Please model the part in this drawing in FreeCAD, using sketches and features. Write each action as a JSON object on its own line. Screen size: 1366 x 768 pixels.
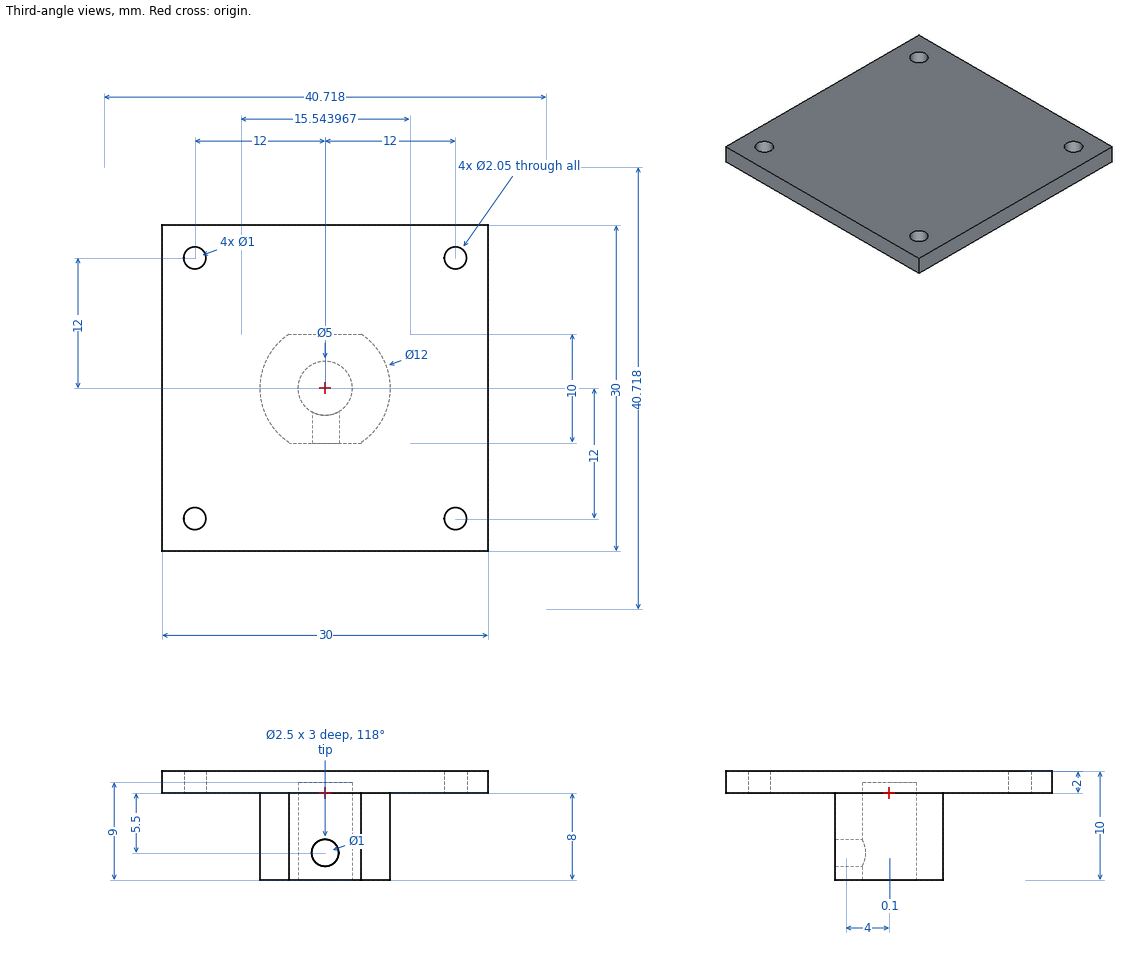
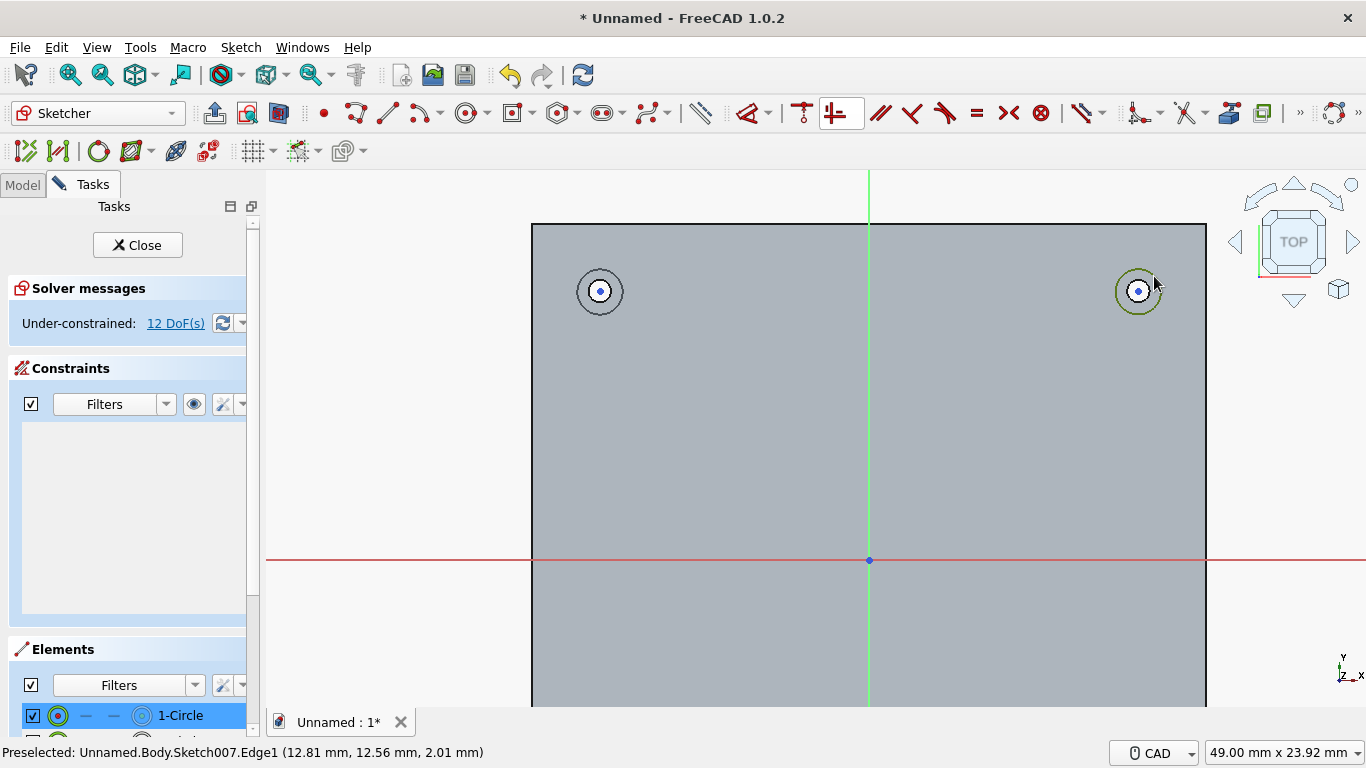
{"action": "scroll", "coordinate": [600, 290], "scroll_direction": "down", "scroll_amount": 3}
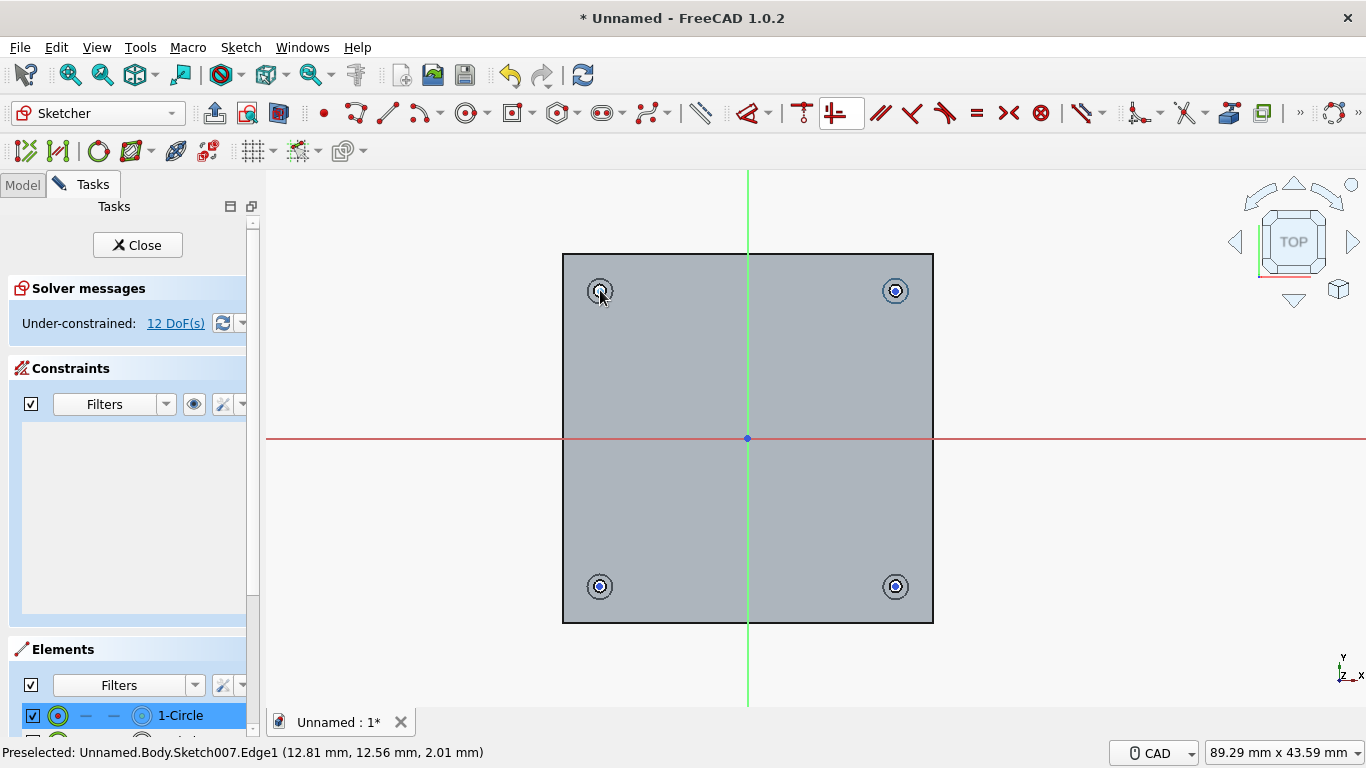
{"action": "left_click", "coordinate": [904, 578]}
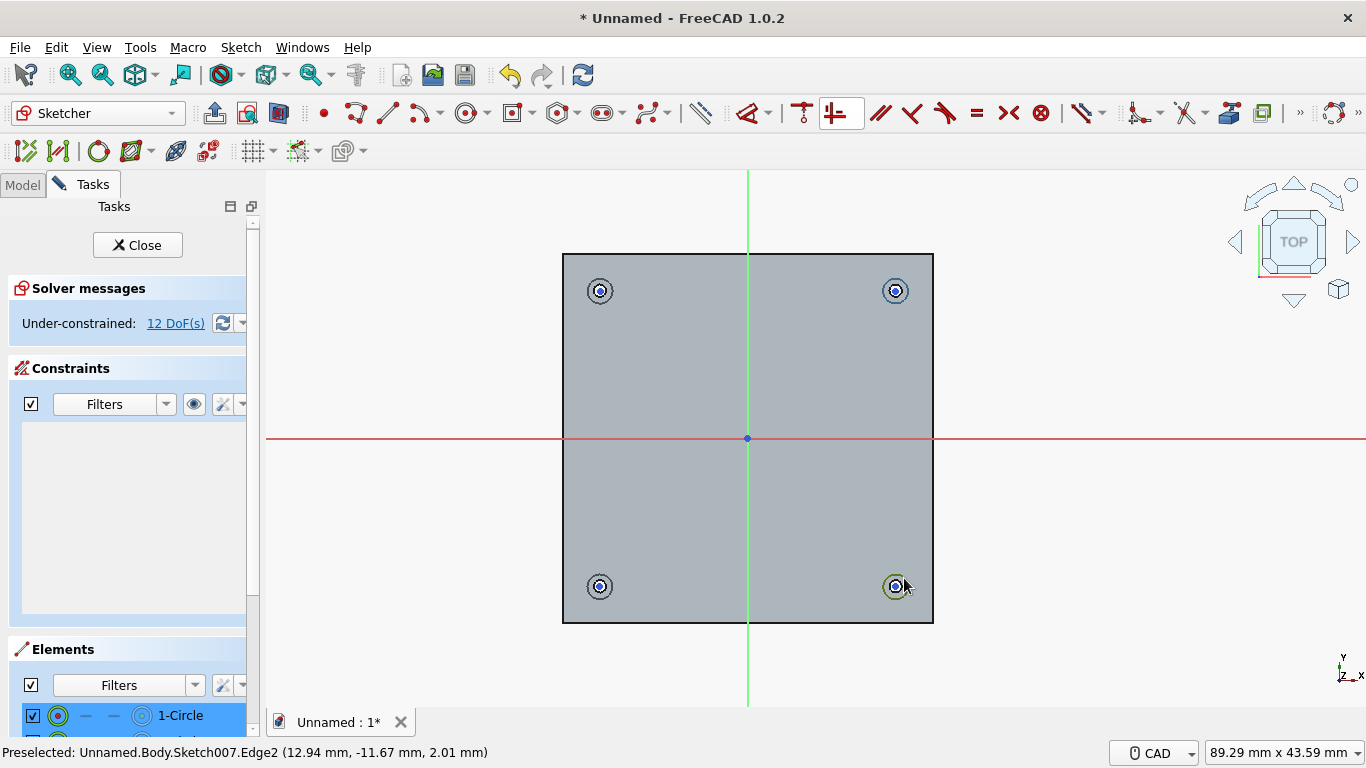
{"action": "left_click", "coordinate": [609, 578]}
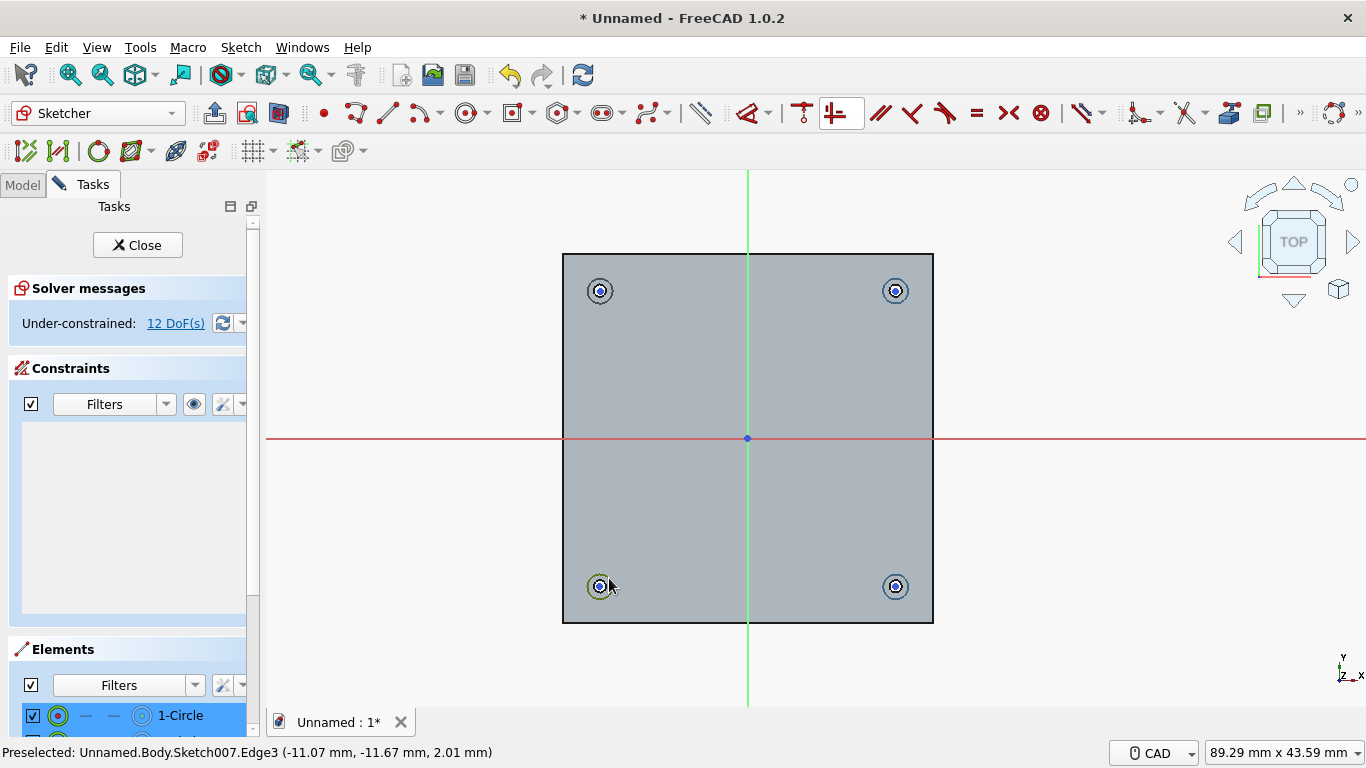
{"action": "left_click", "coordinate": [609, 282]}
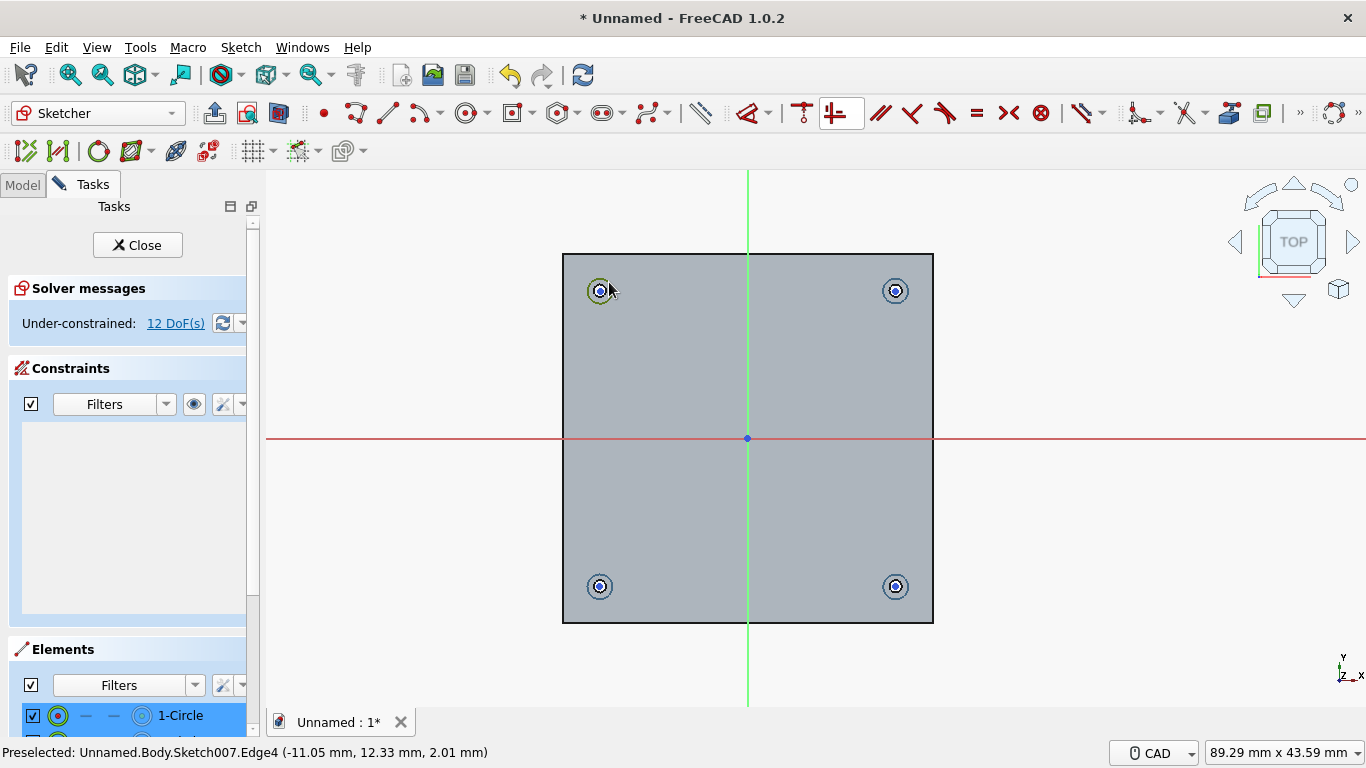
{"action": "key", "text": "e"}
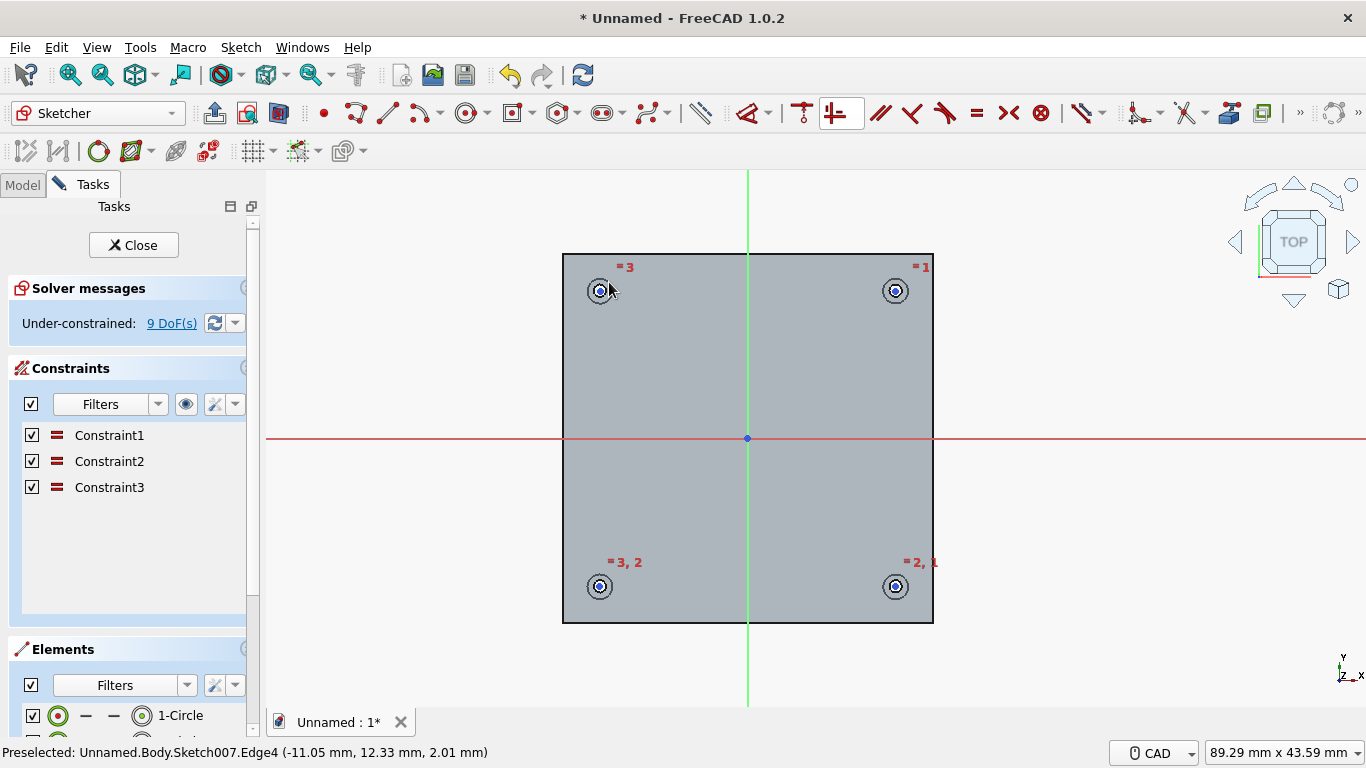
{"action": "left_click", "coordinate": [896, 291]}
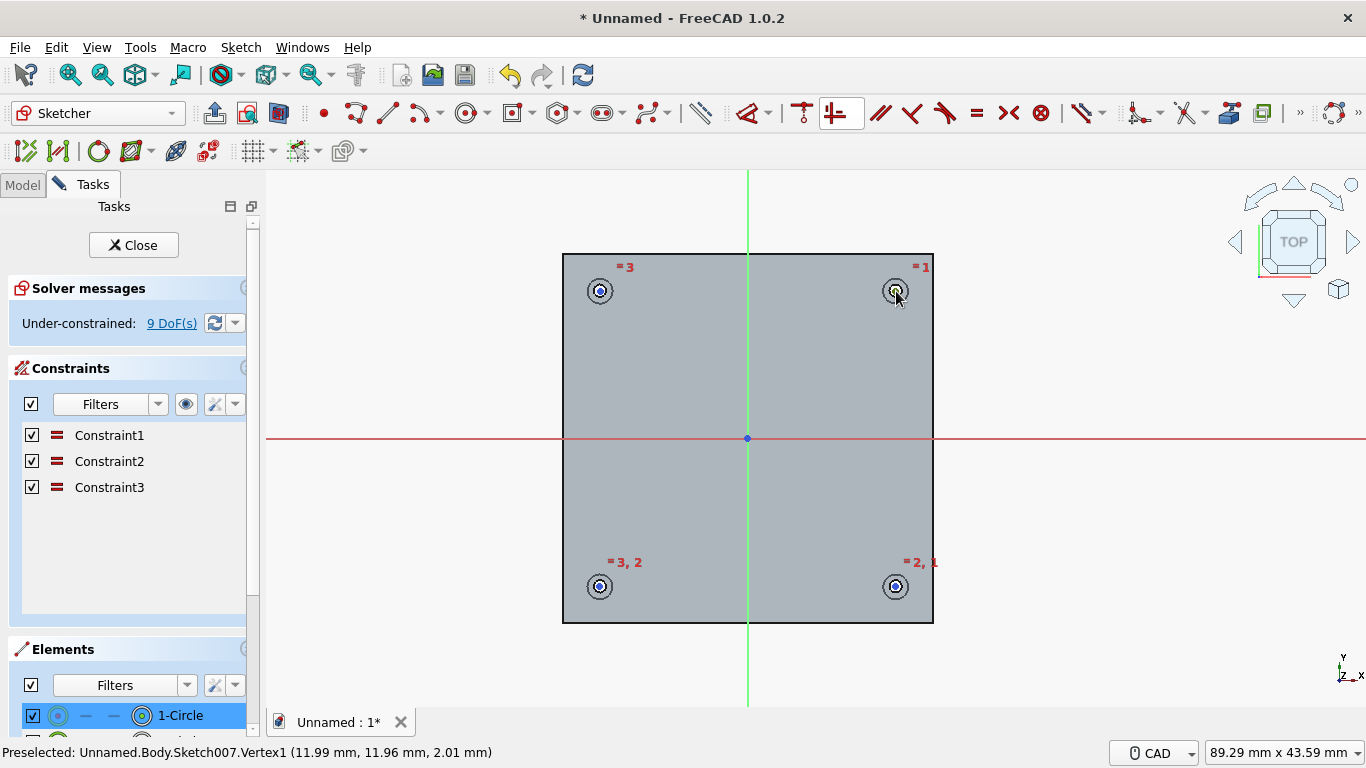
{"action": "left_click", "coordinate": [896, 587]}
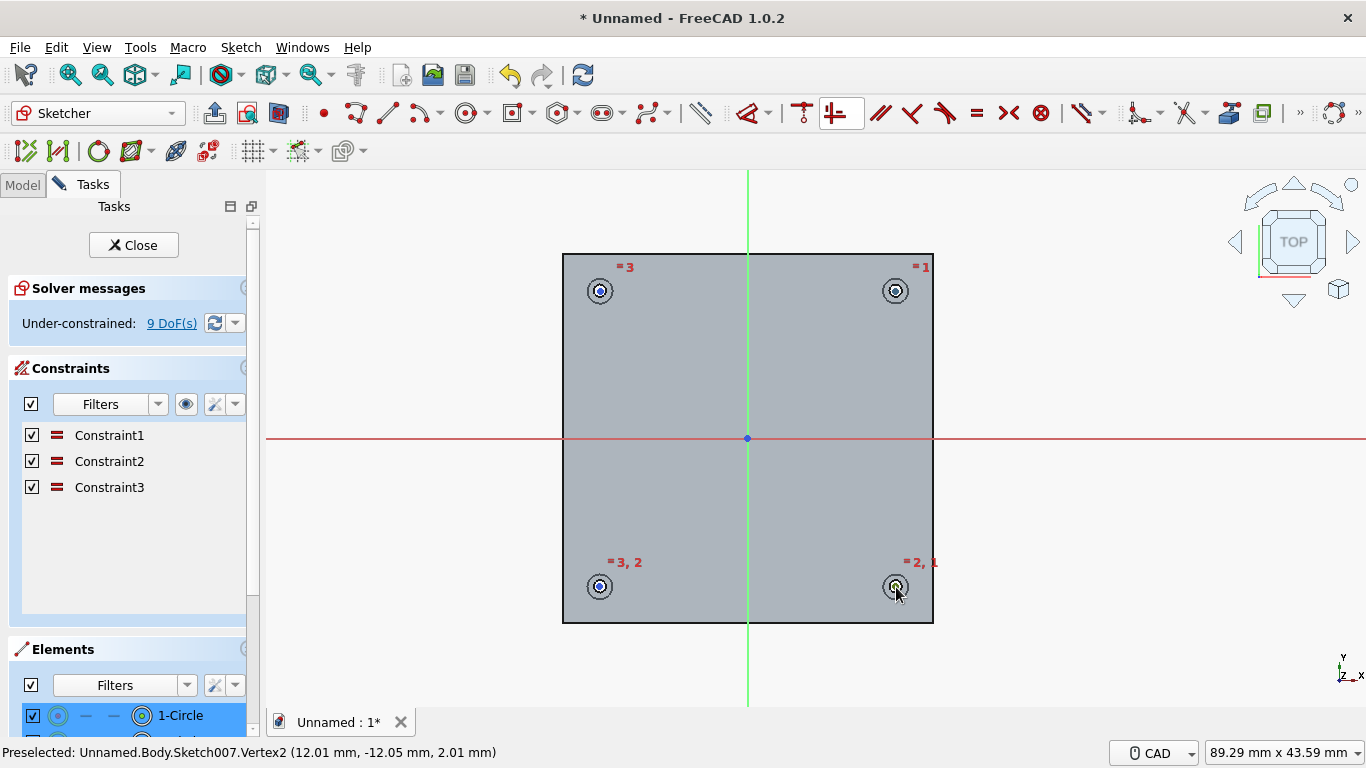
{"action": "key", "text": "v"}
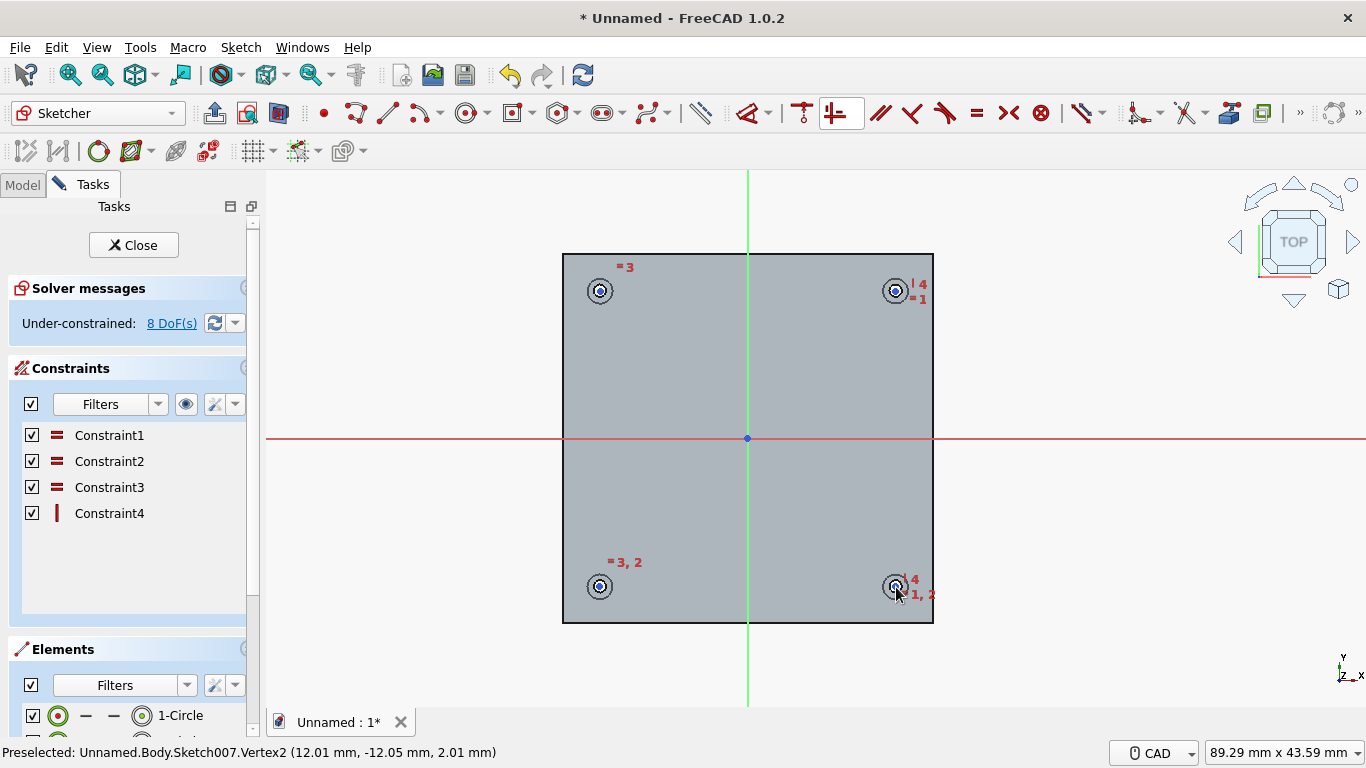
{"action": "left_click", "coordinate": [896, 587]}